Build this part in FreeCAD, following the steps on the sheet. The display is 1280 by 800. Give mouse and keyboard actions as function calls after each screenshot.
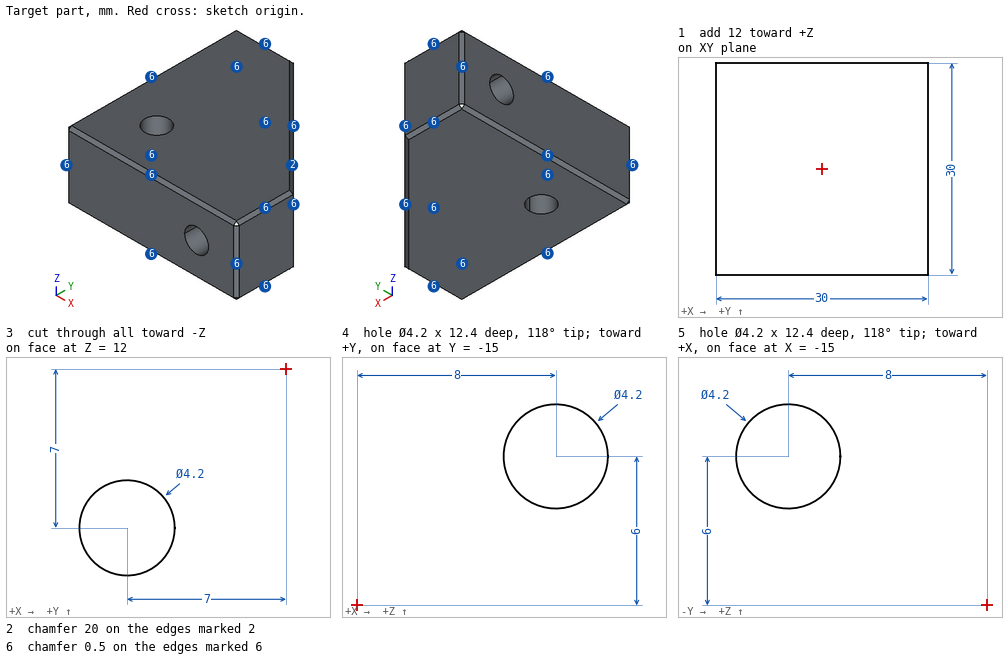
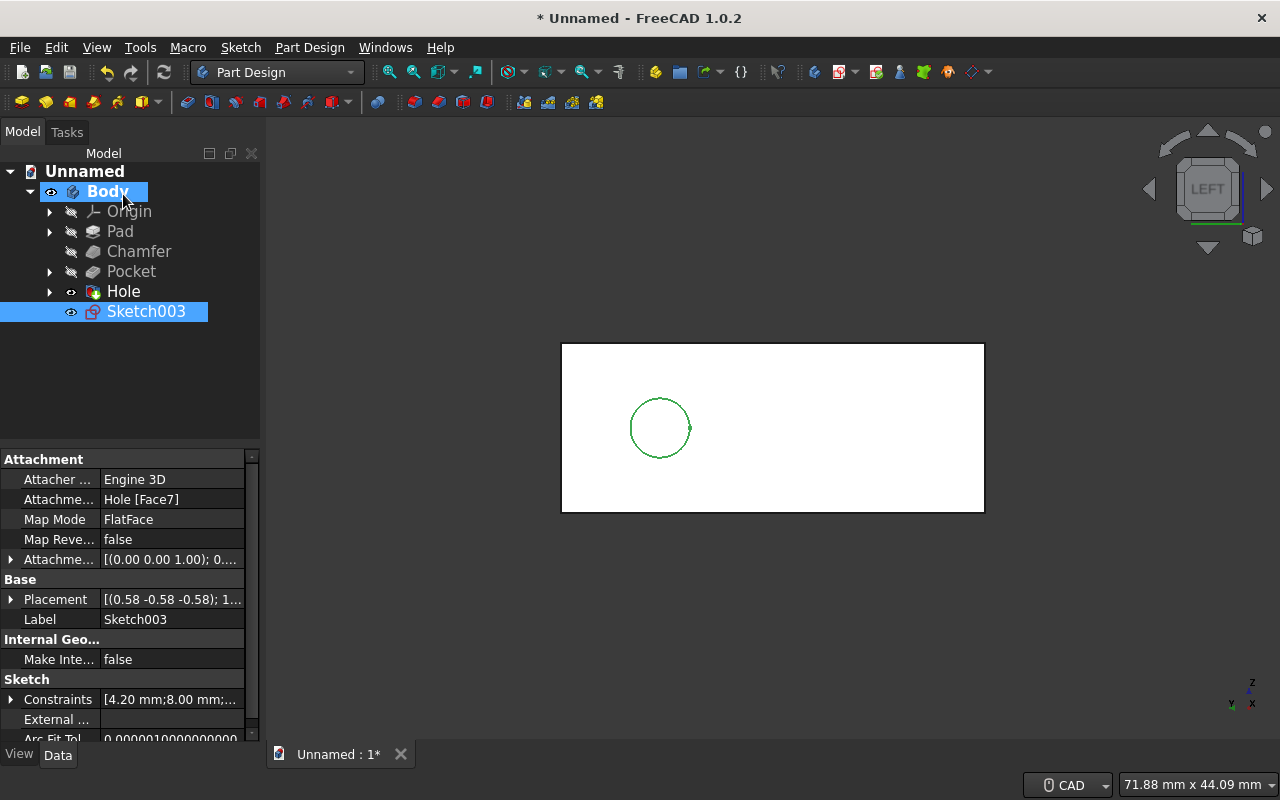
click(212, 102)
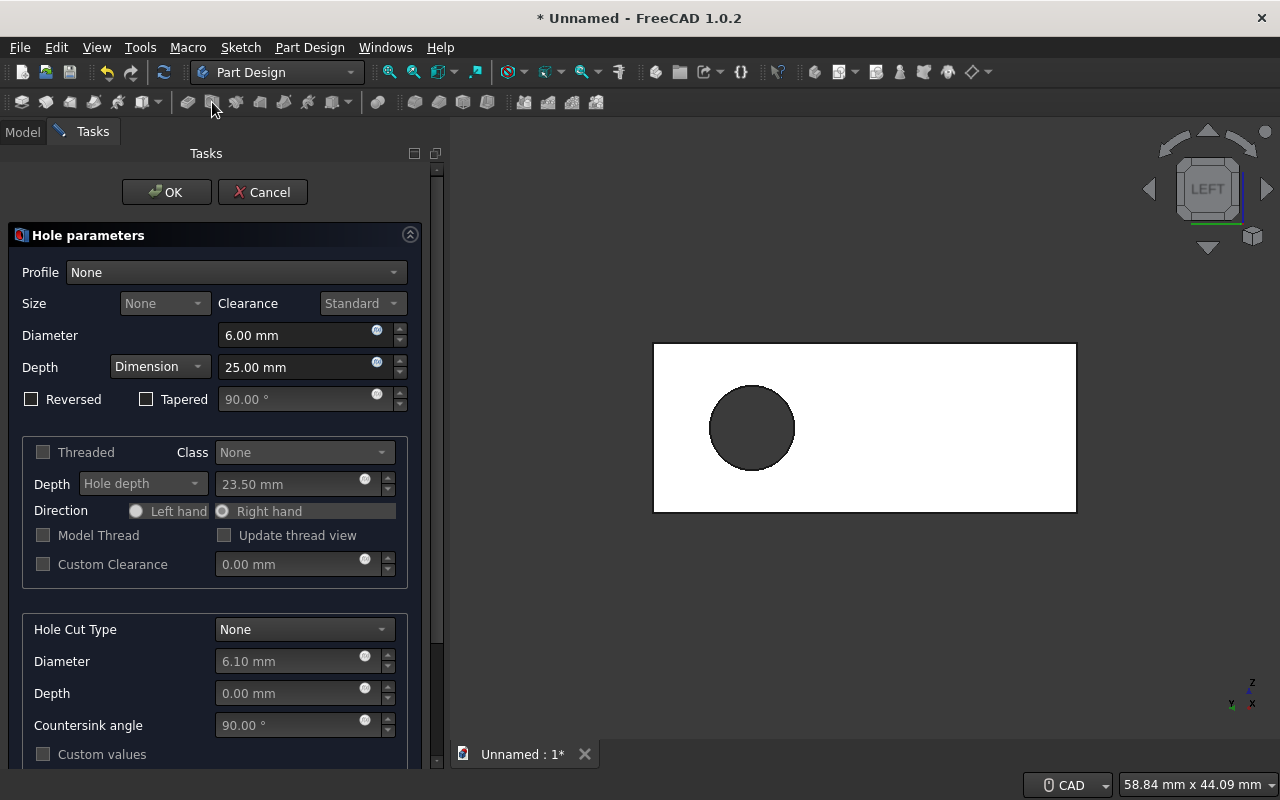
triple_click(305, 335)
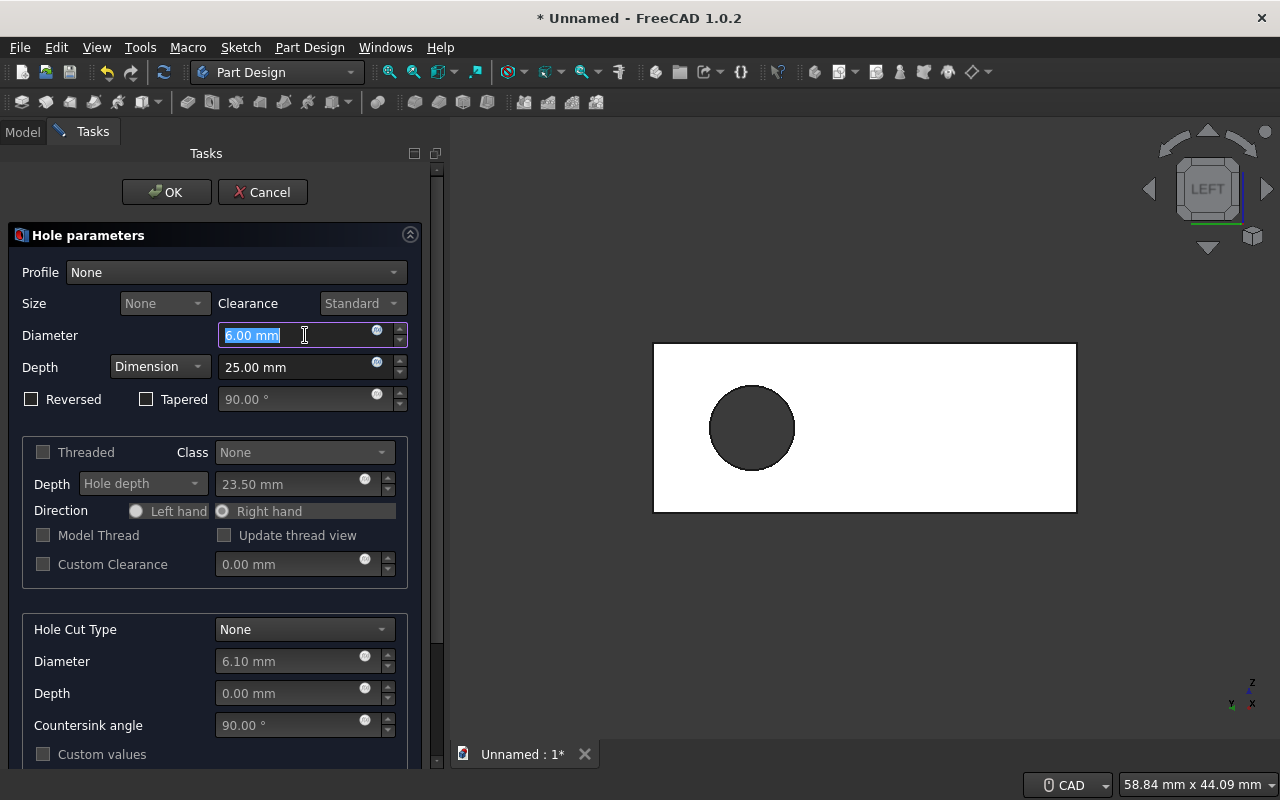
text(4.2)
key(Tab)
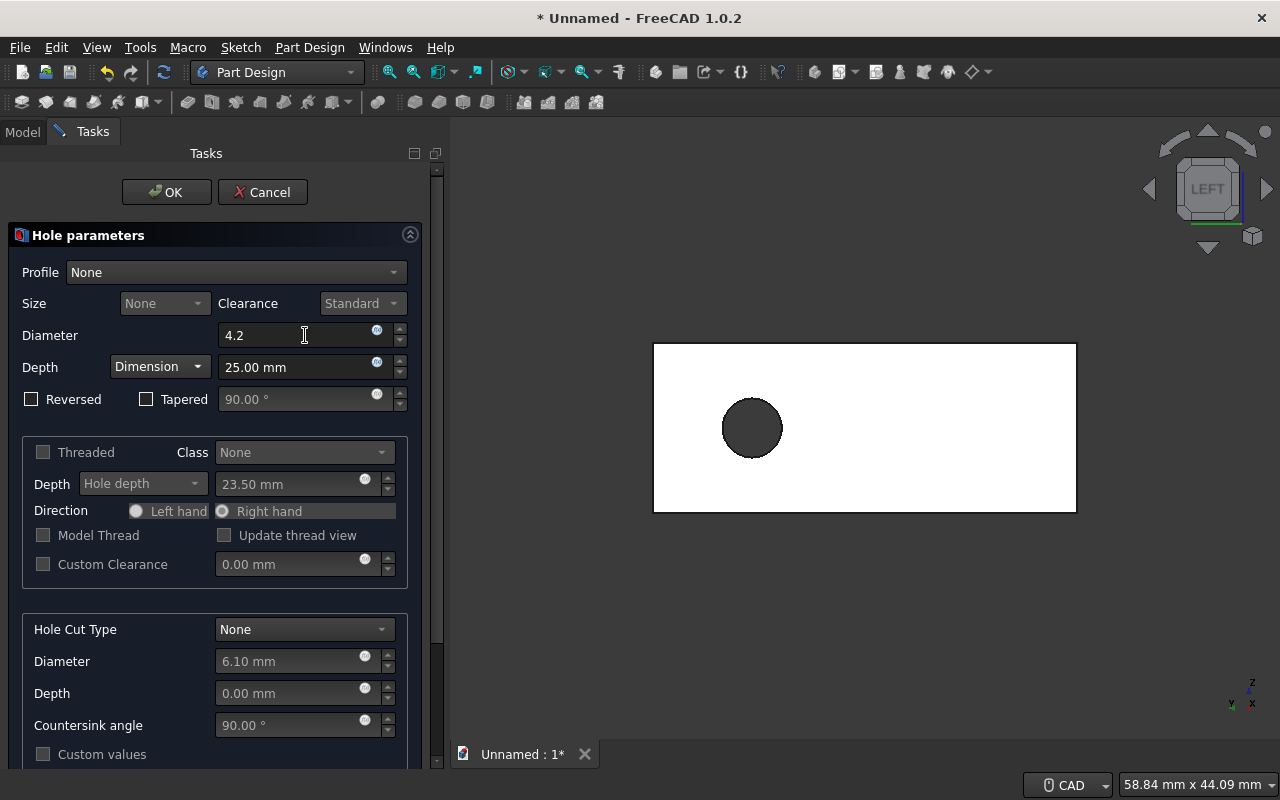
triple_click(305, 367)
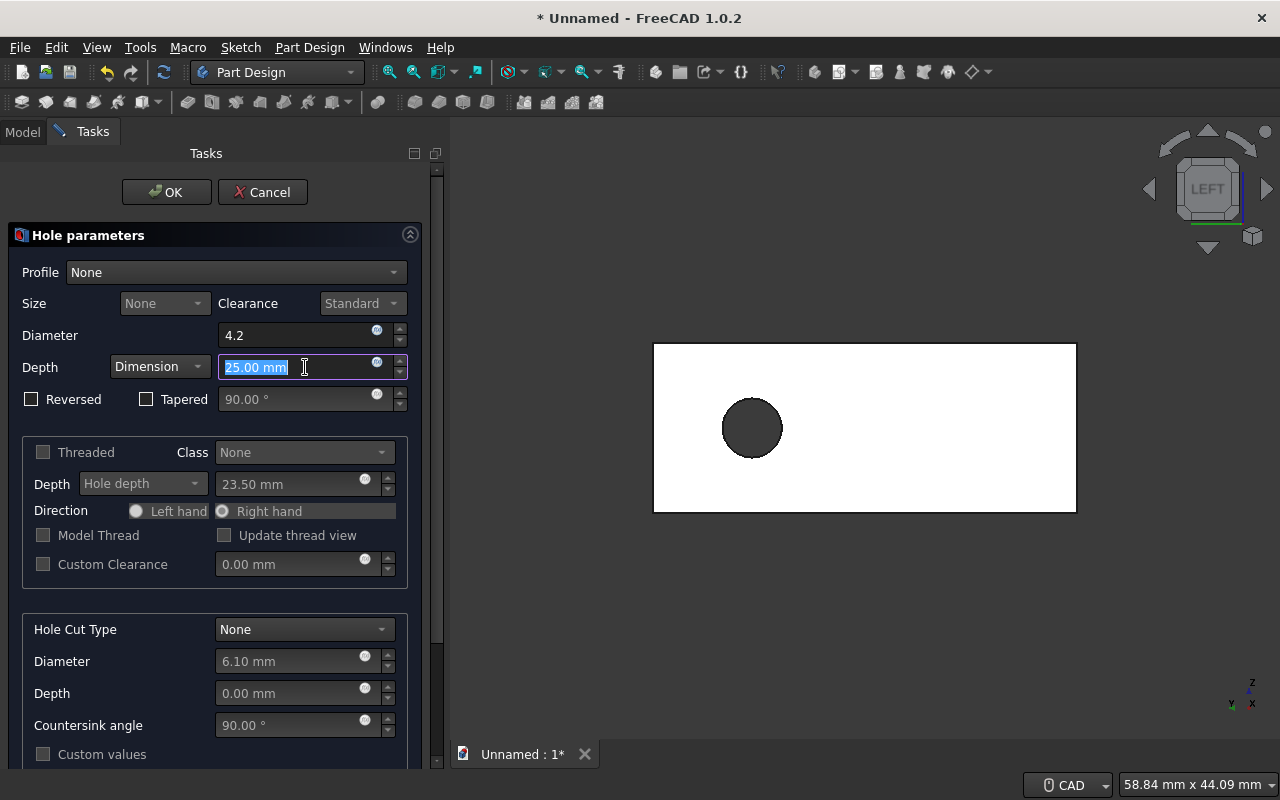
text(12.4)
key(Tab)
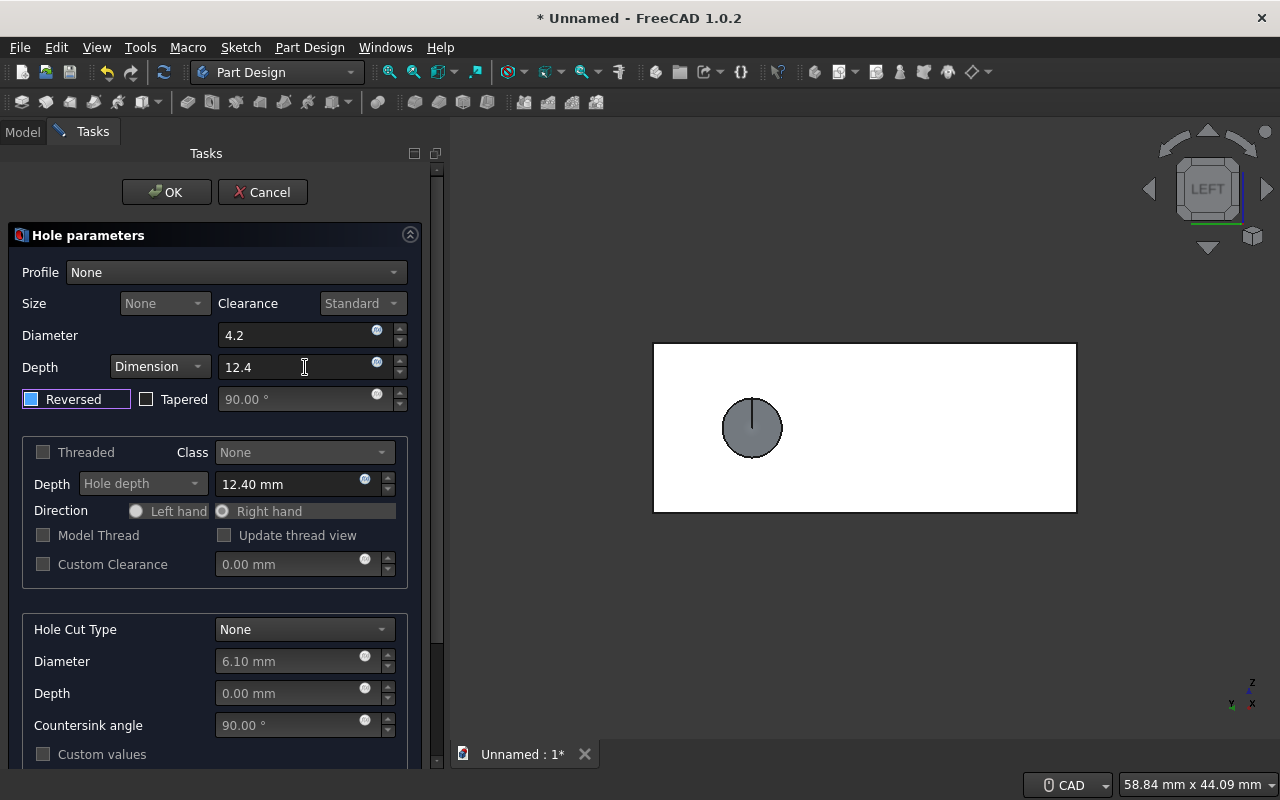
click(167, 192)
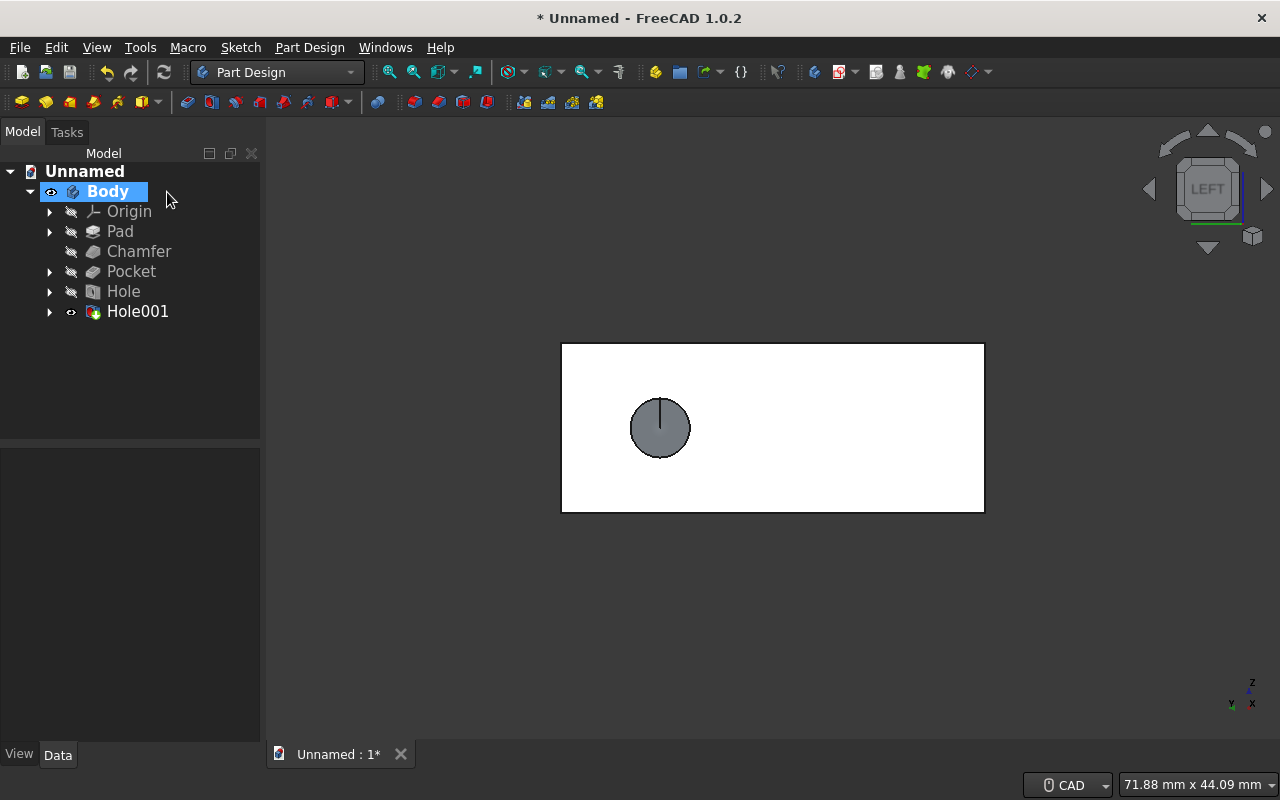
click(390, 72)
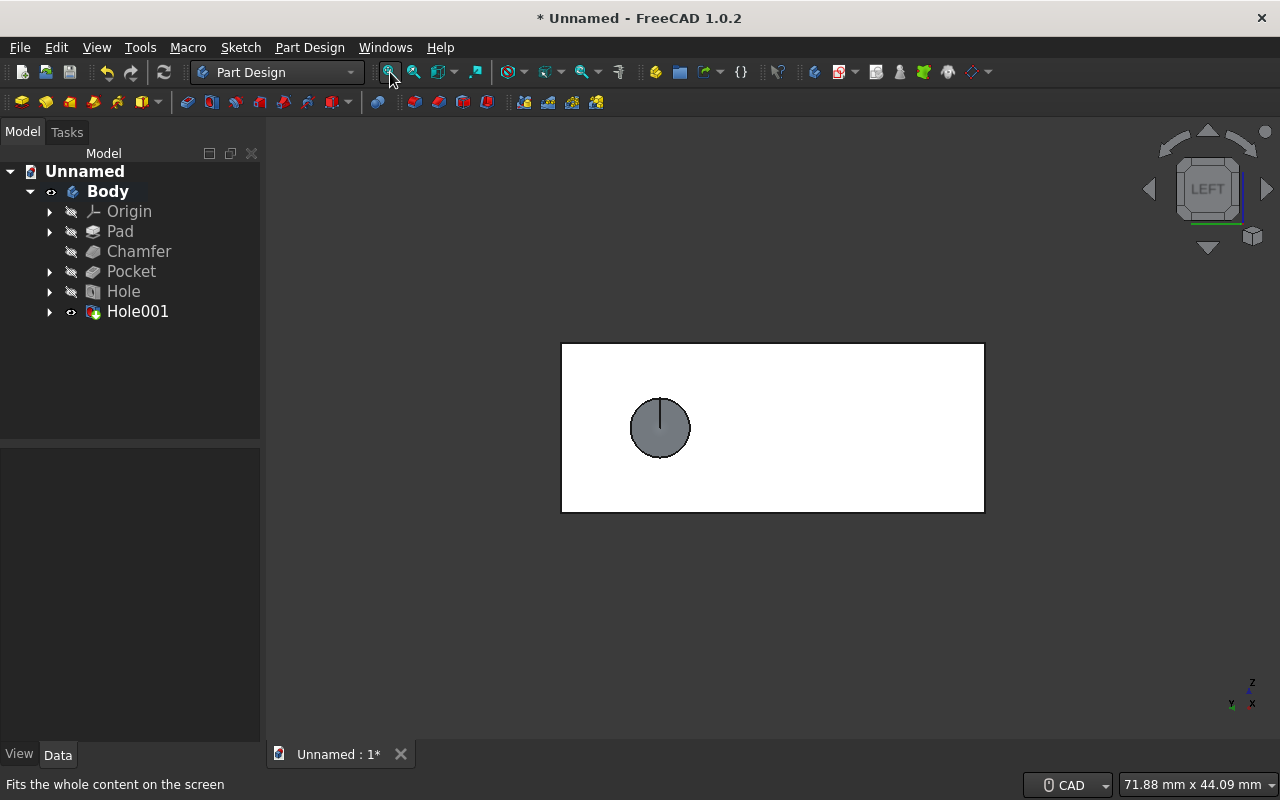
click(773, 342)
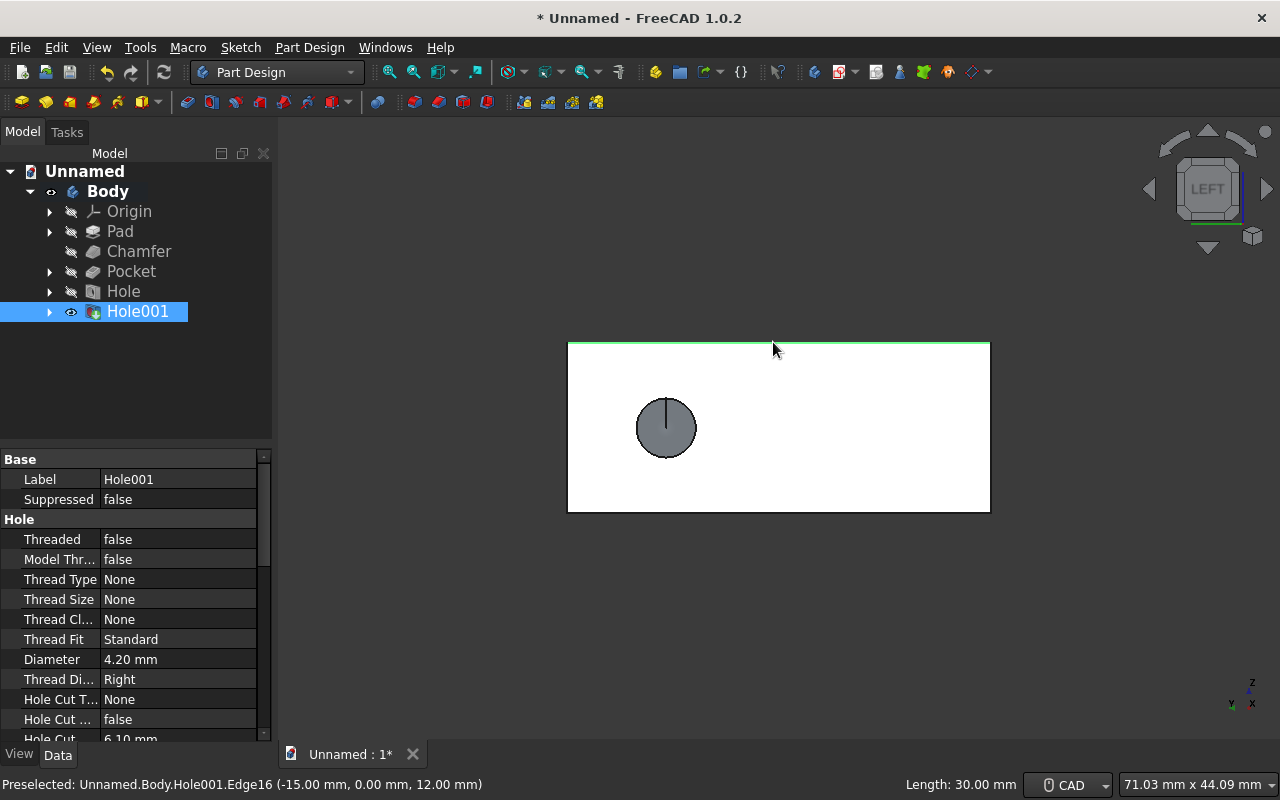
click(779, 512, ctrl)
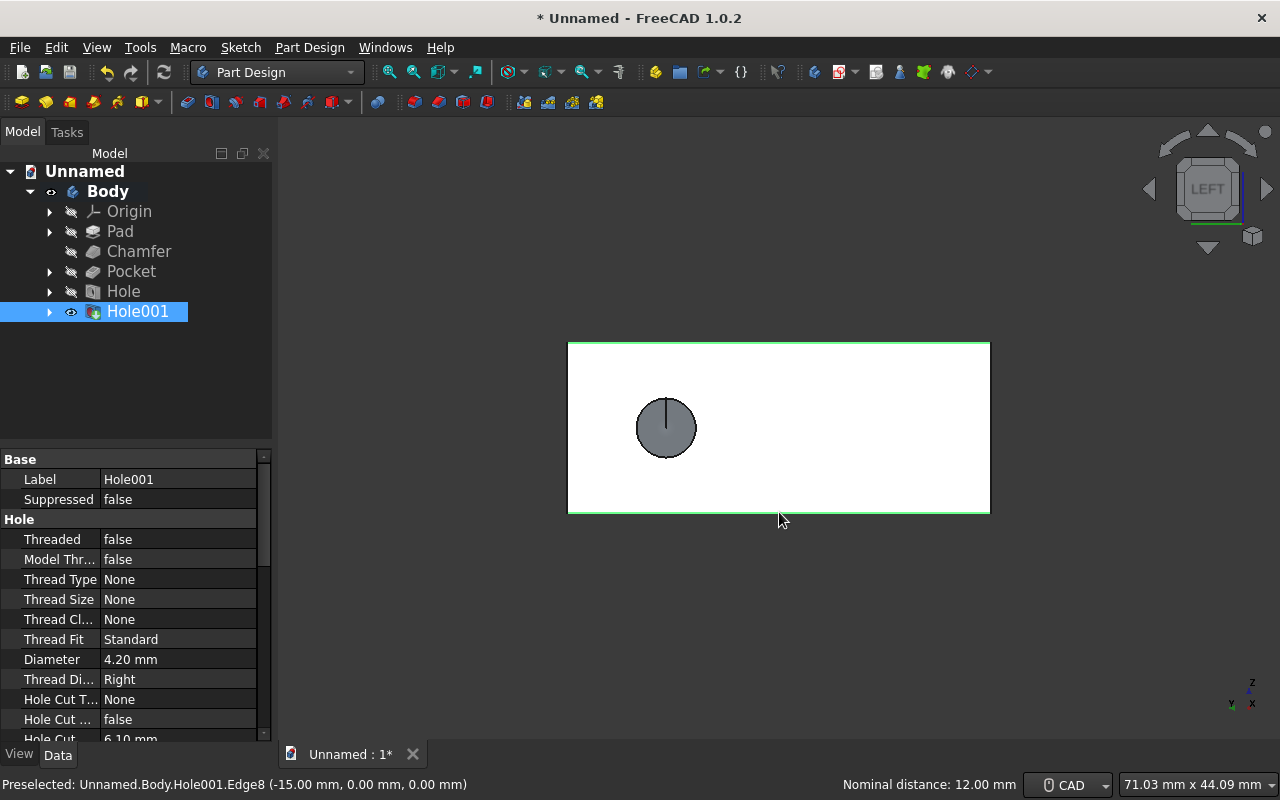
click(991, 427, ctrl)